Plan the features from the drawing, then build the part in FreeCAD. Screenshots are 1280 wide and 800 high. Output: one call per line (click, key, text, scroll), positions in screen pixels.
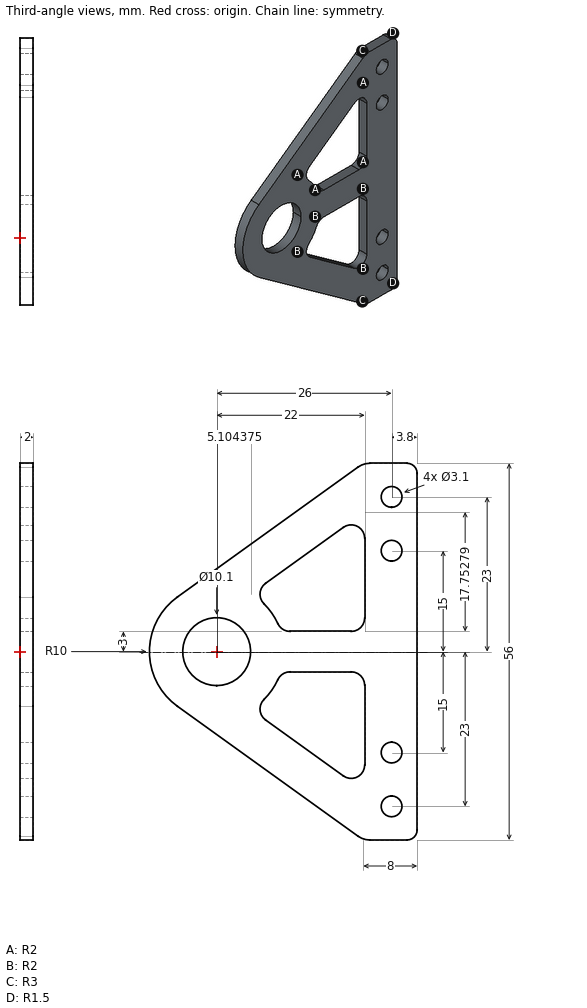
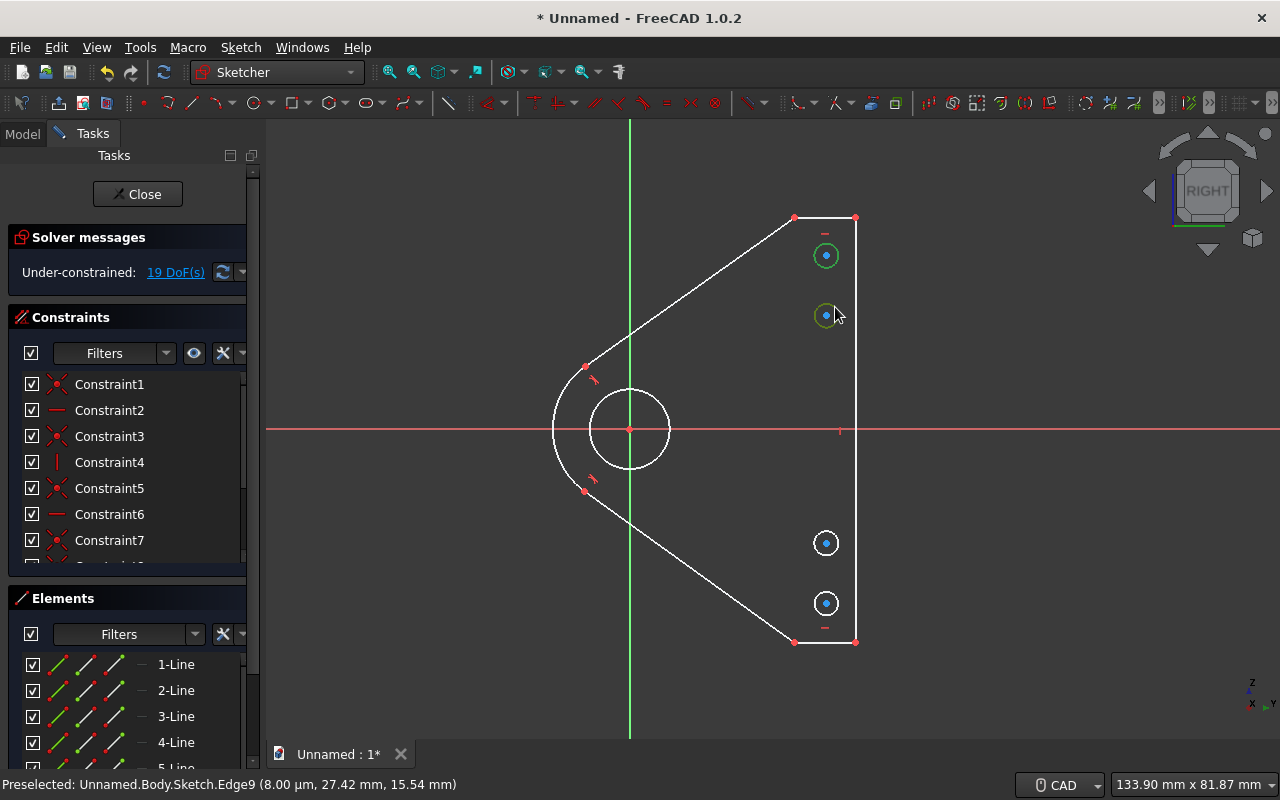
click(835, 535)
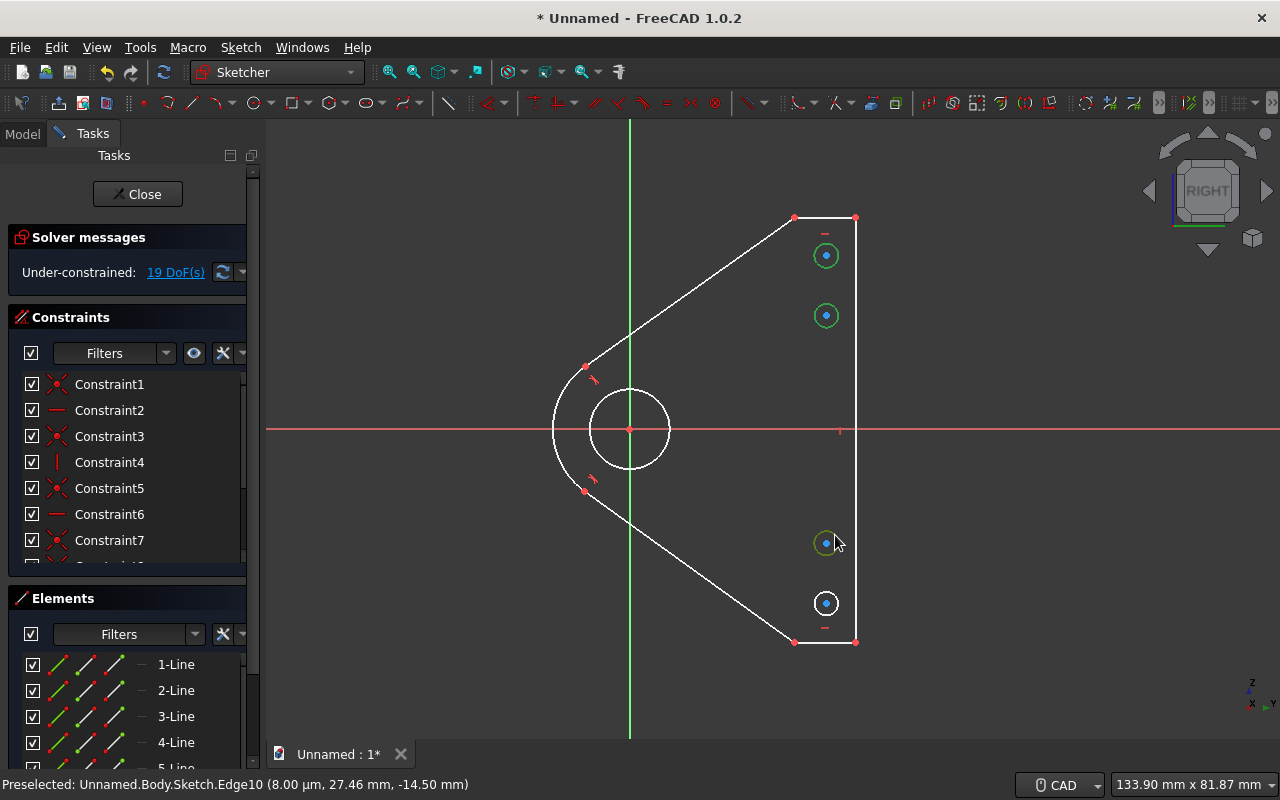
click(835, 595)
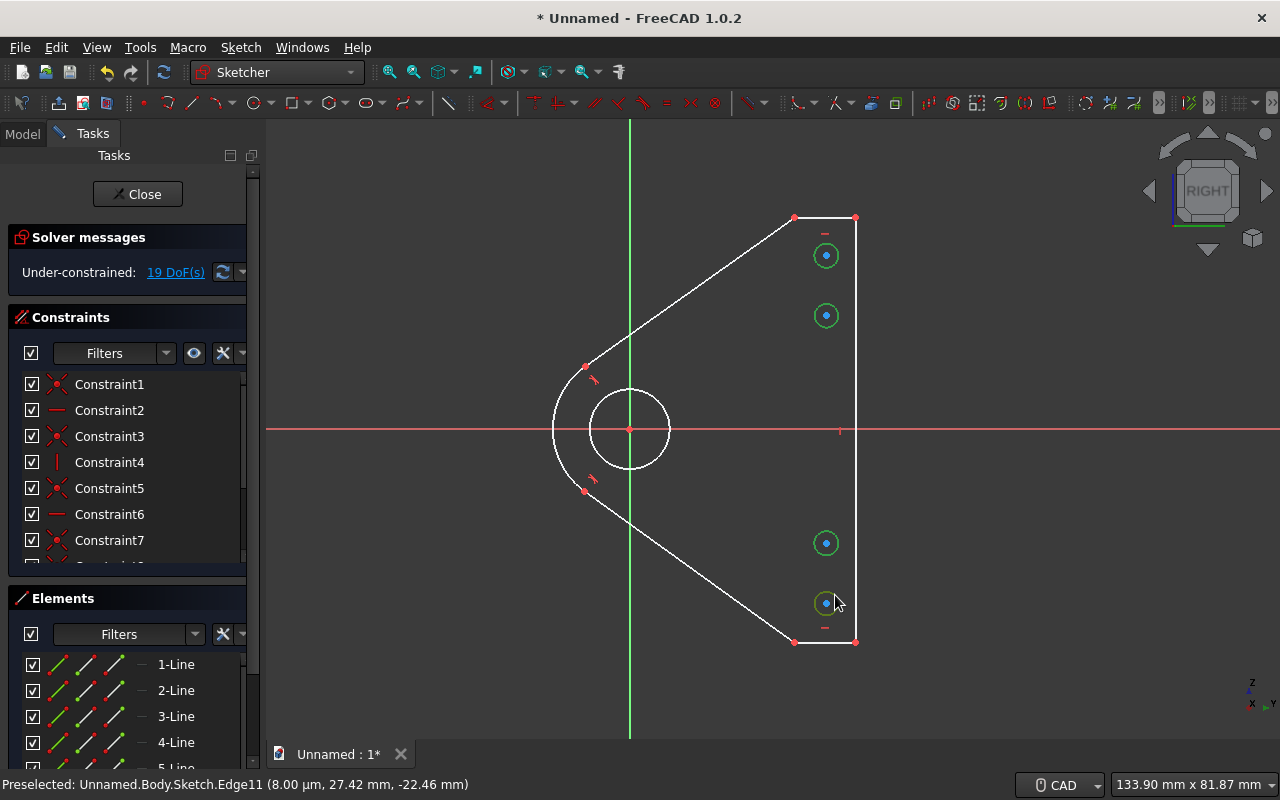
click(668, 104)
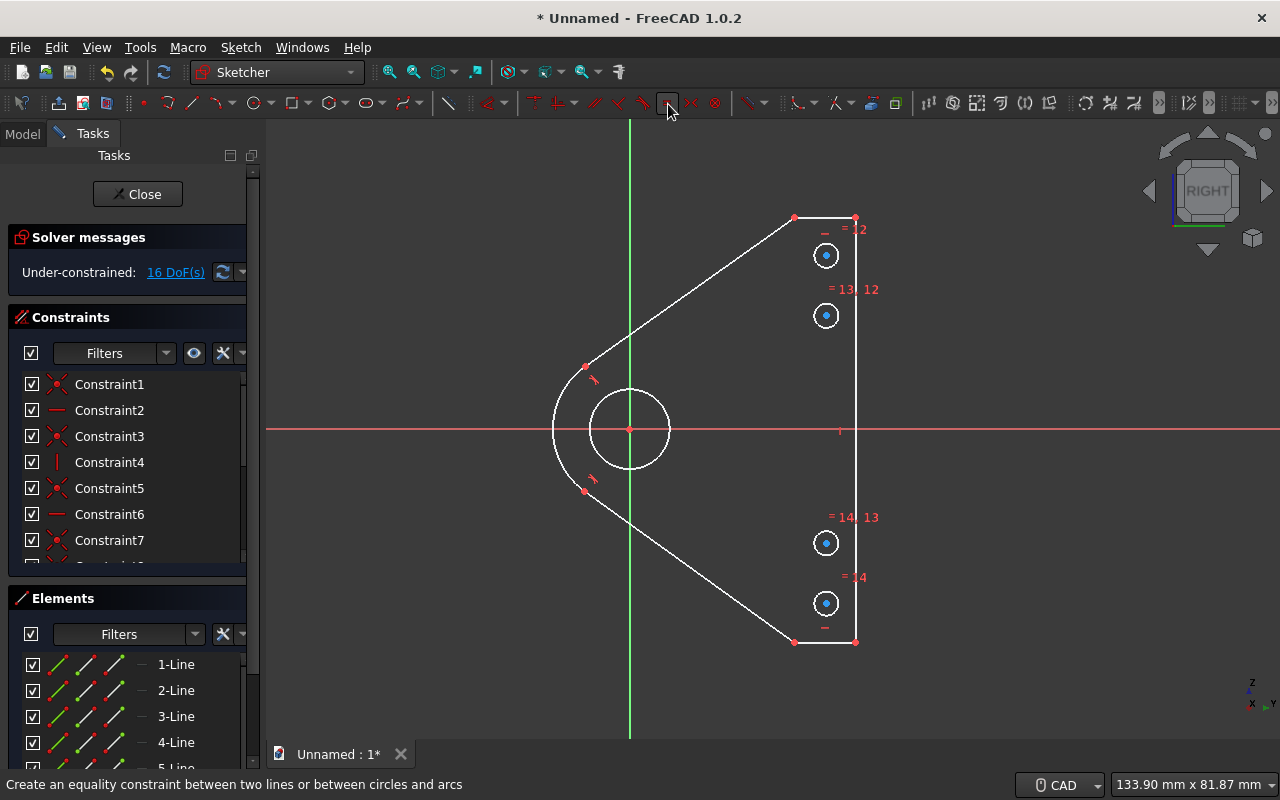
click(826, 256)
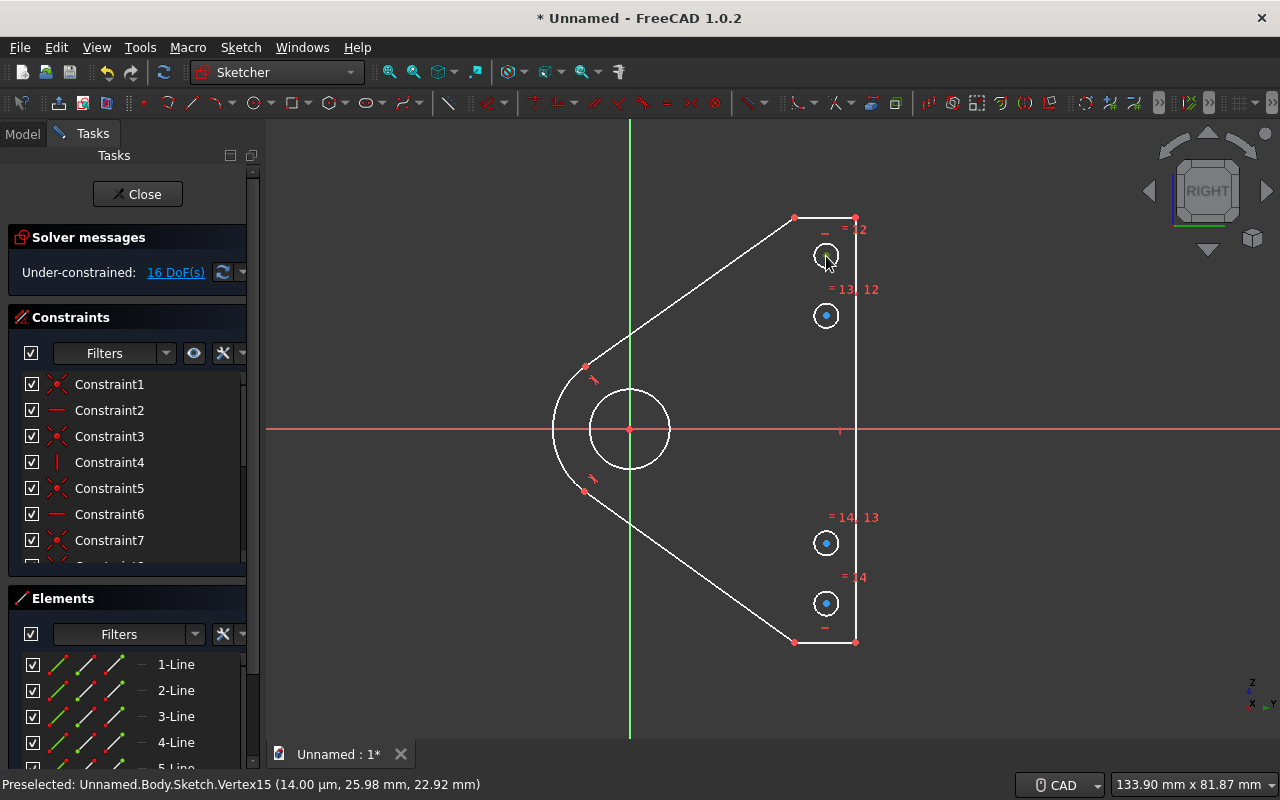
click(826, 316)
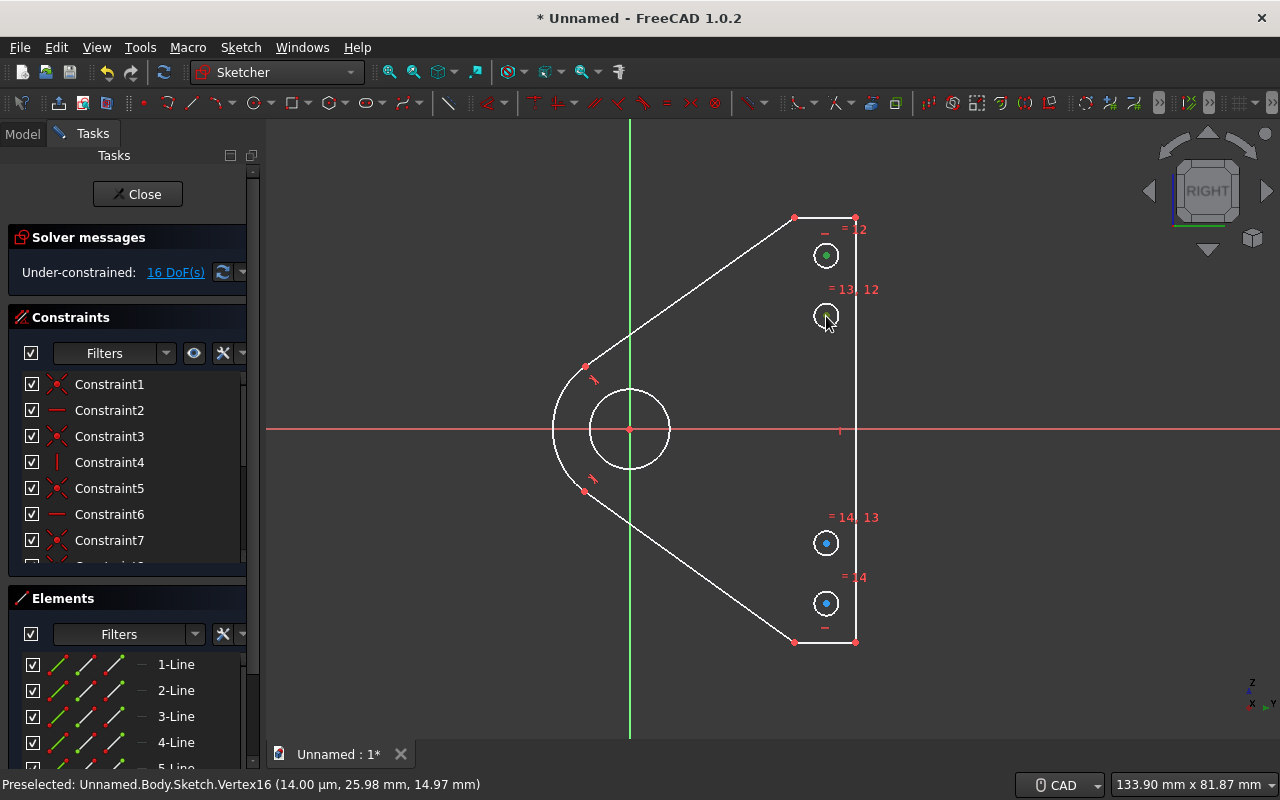
key(v)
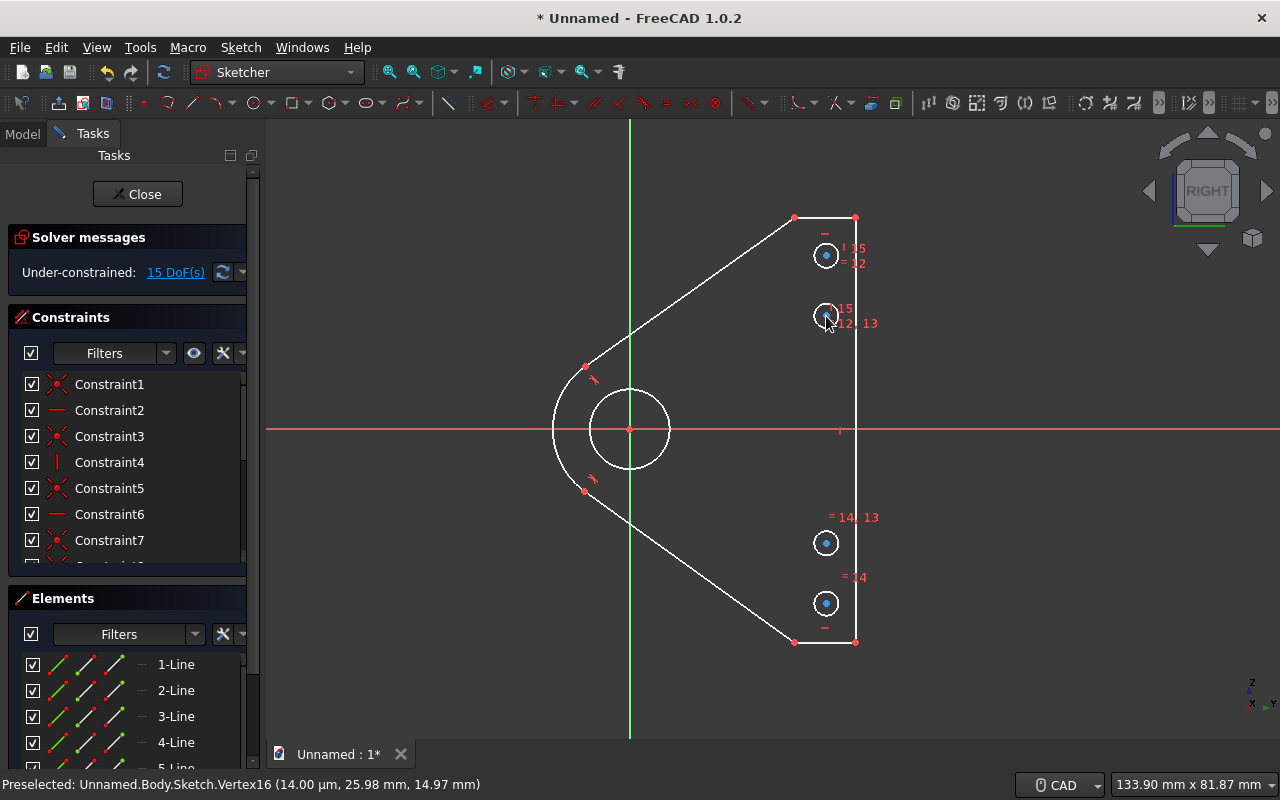
click(824, 318)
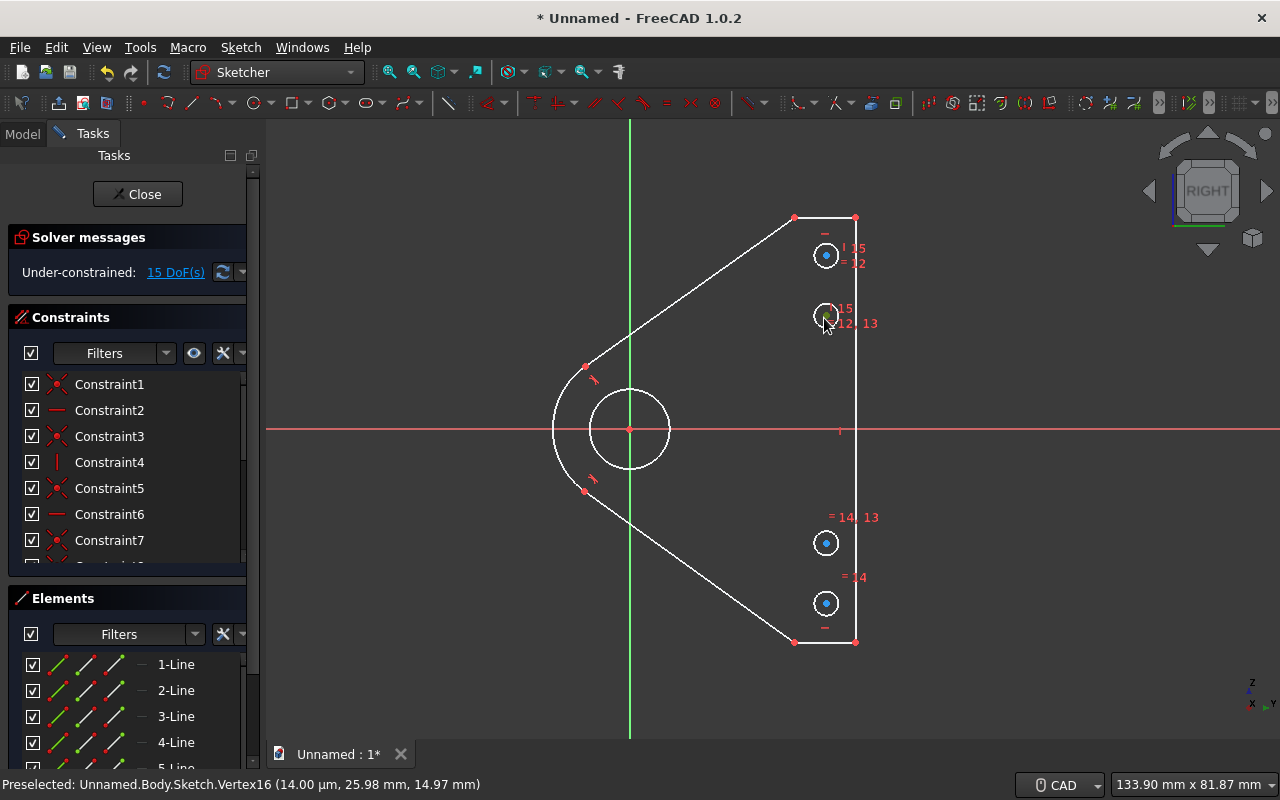
click(826, 543)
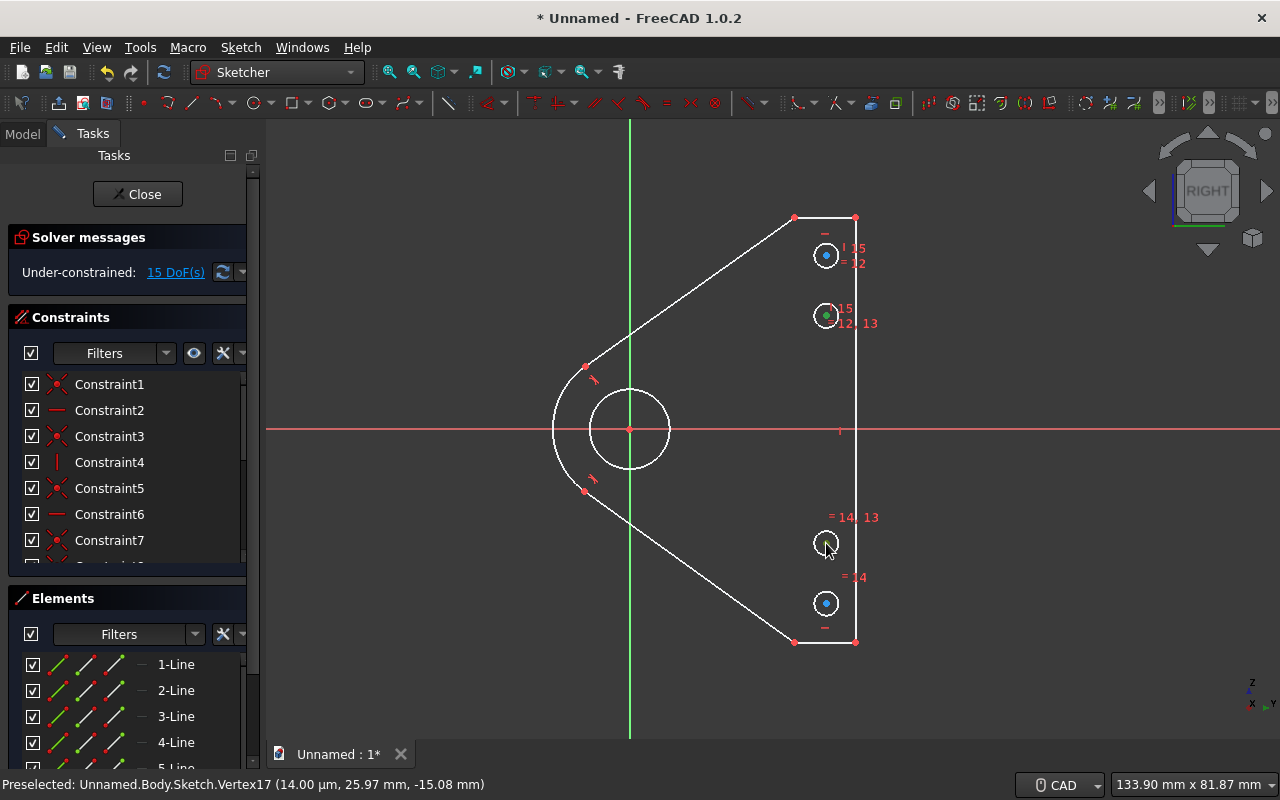
key(v)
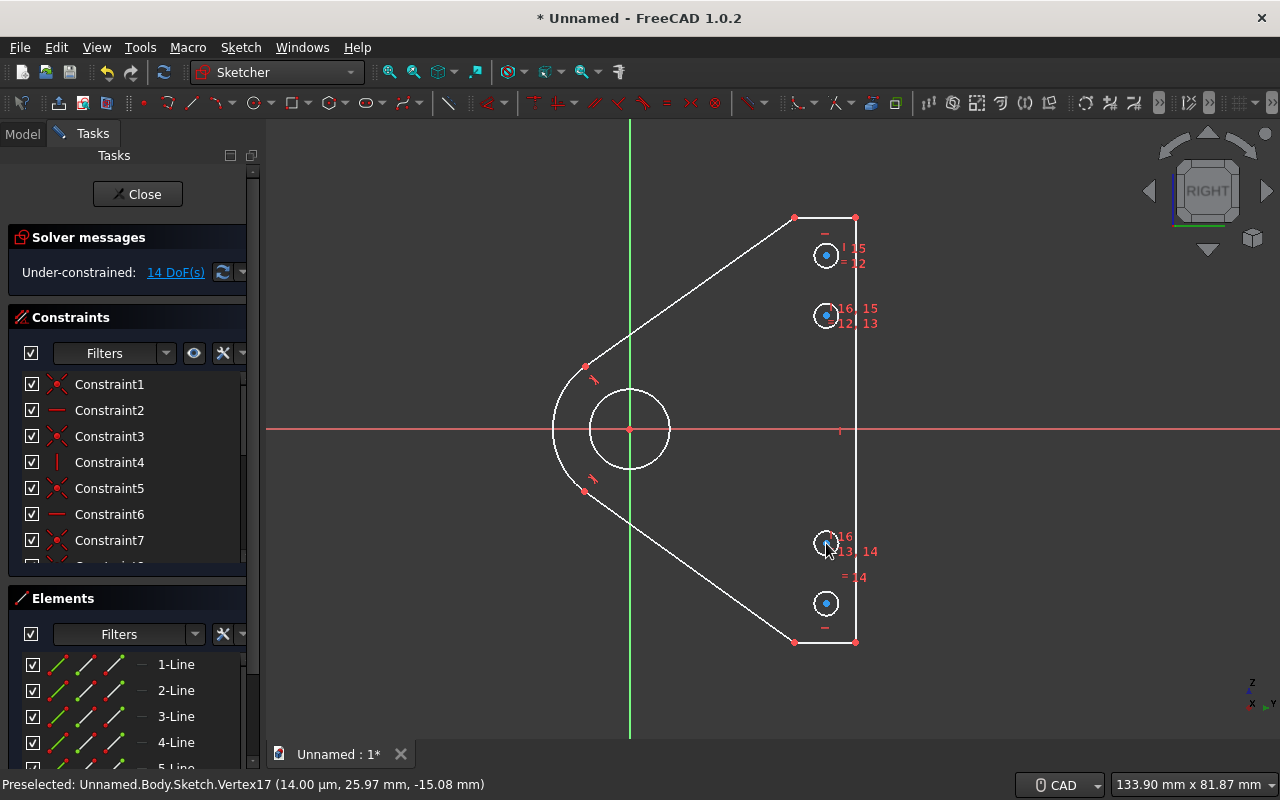
click(824, 545)